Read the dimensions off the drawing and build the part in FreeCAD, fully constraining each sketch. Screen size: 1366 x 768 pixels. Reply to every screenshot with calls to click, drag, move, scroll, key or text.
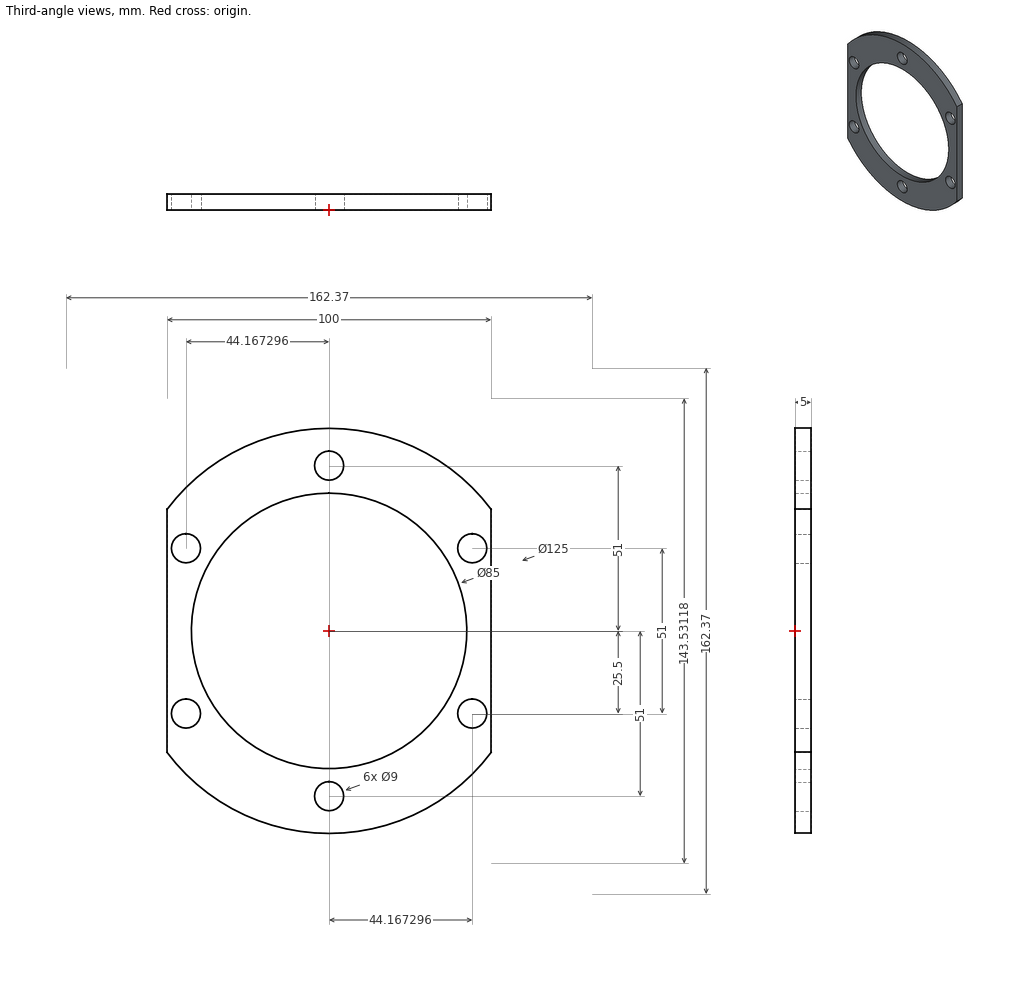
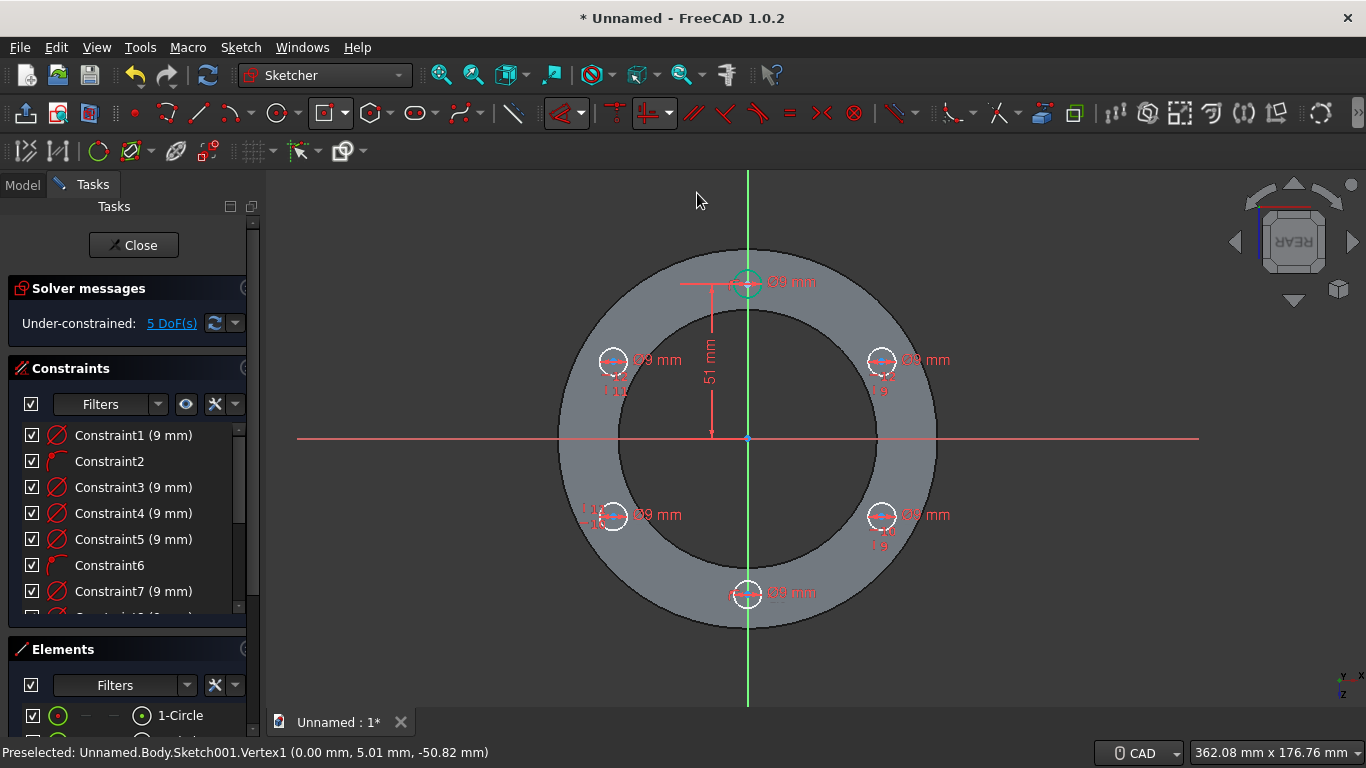
click(748, 595)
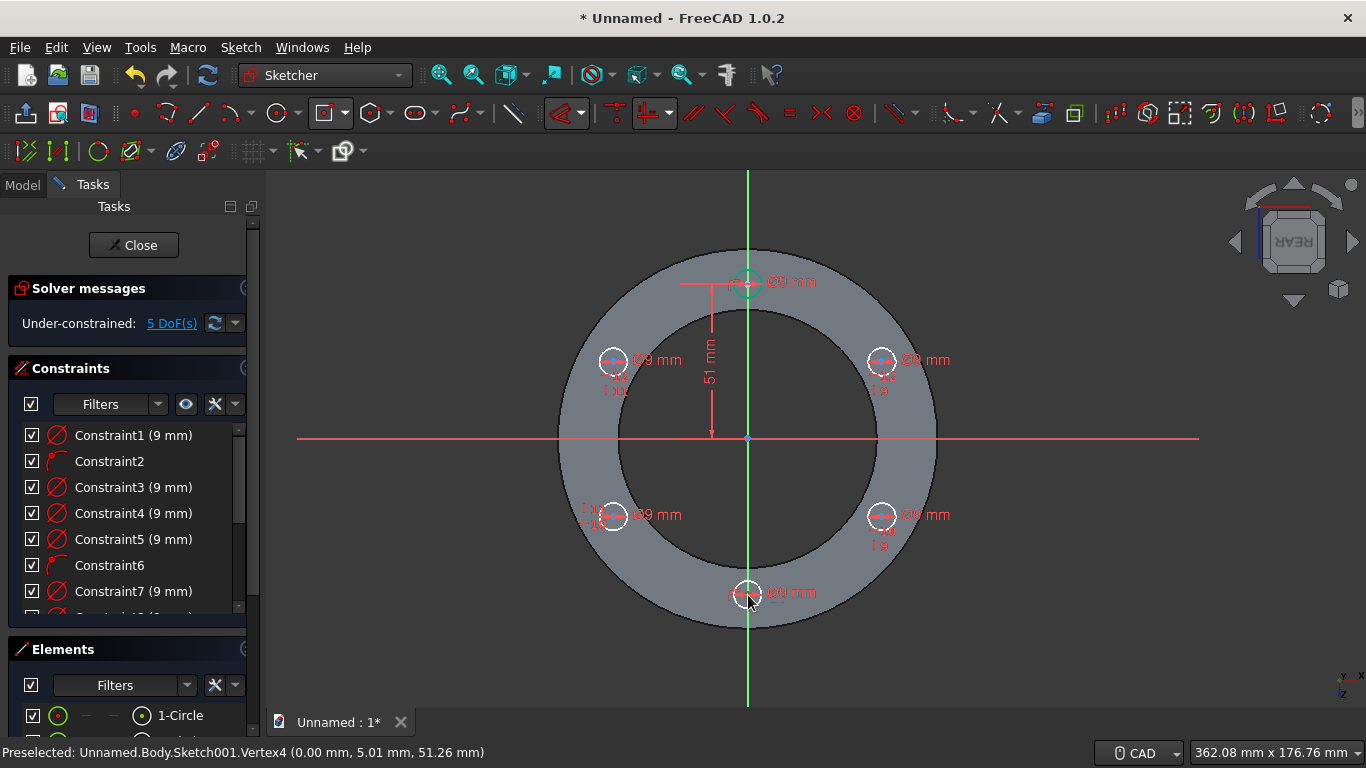
click(584, 114)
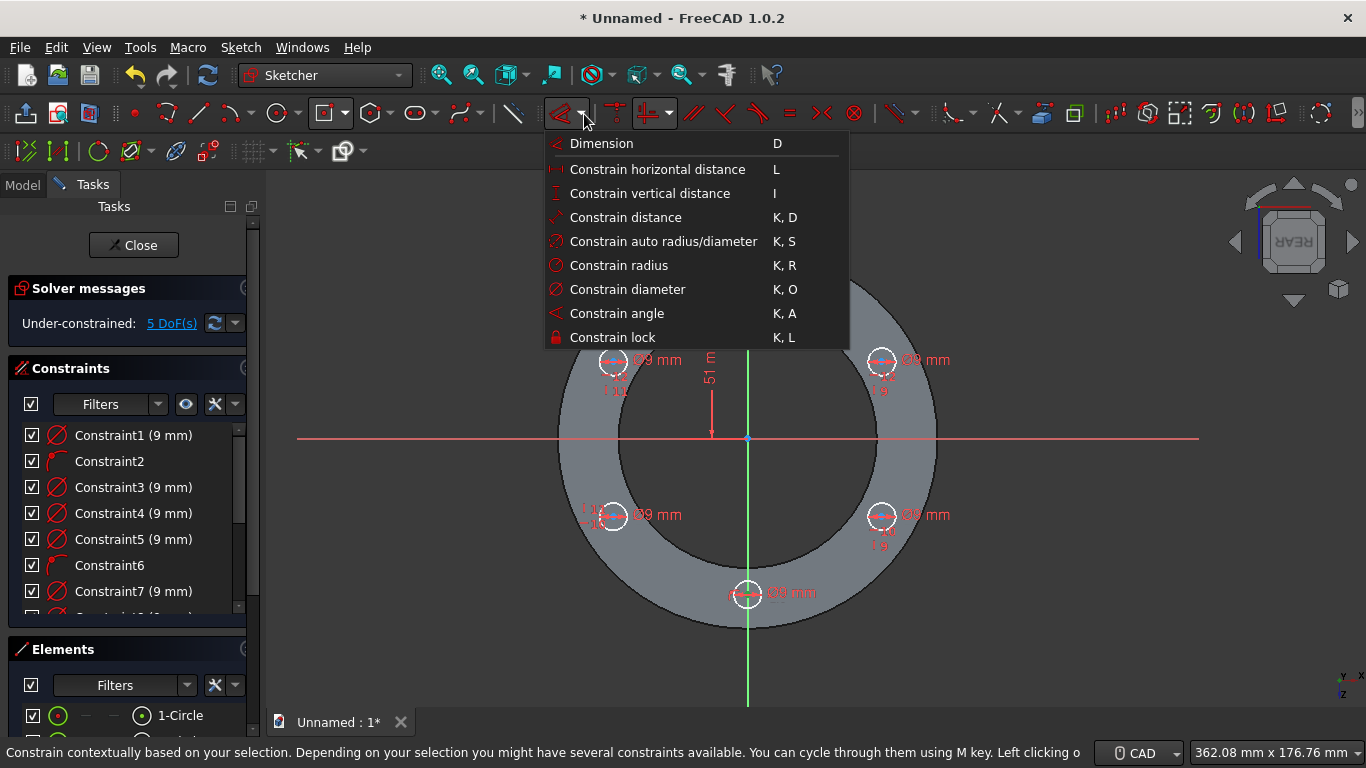
click(697, 193)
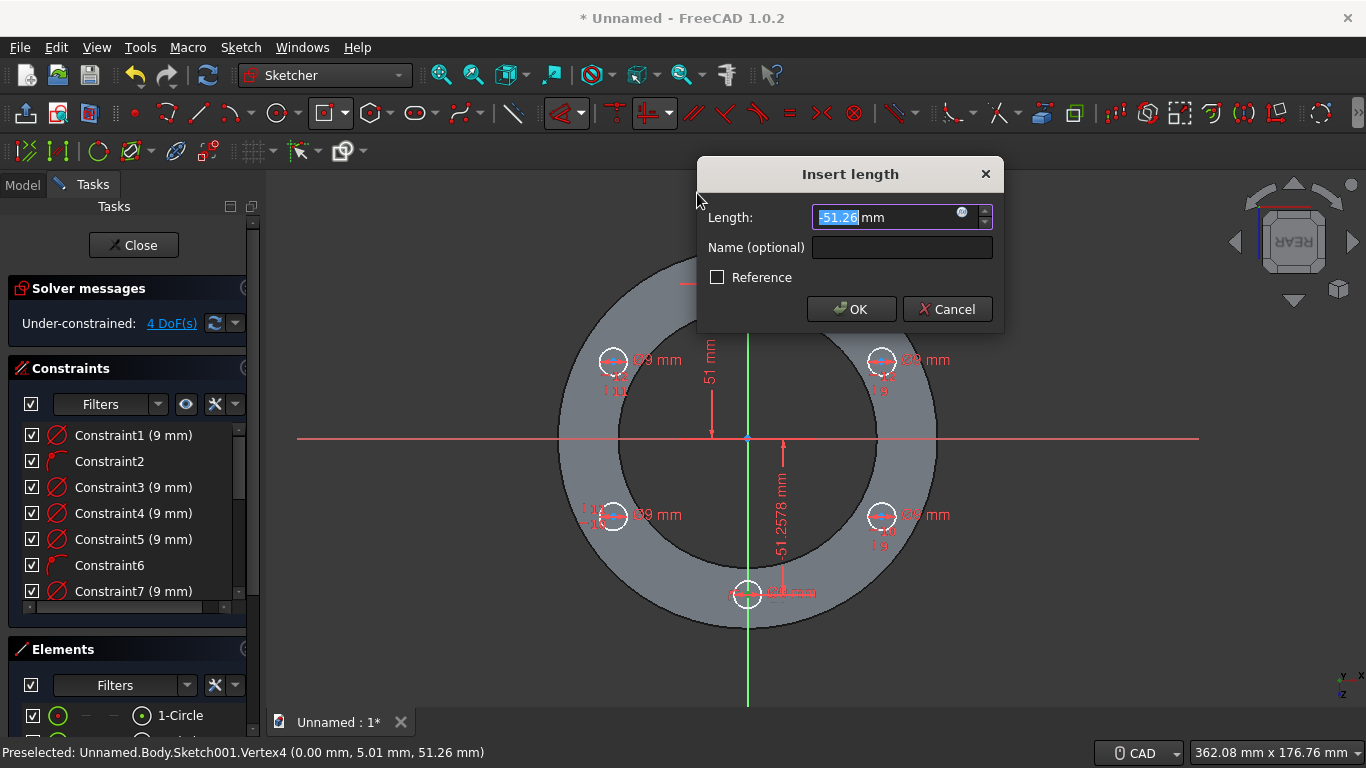
text(-51)
key(Return)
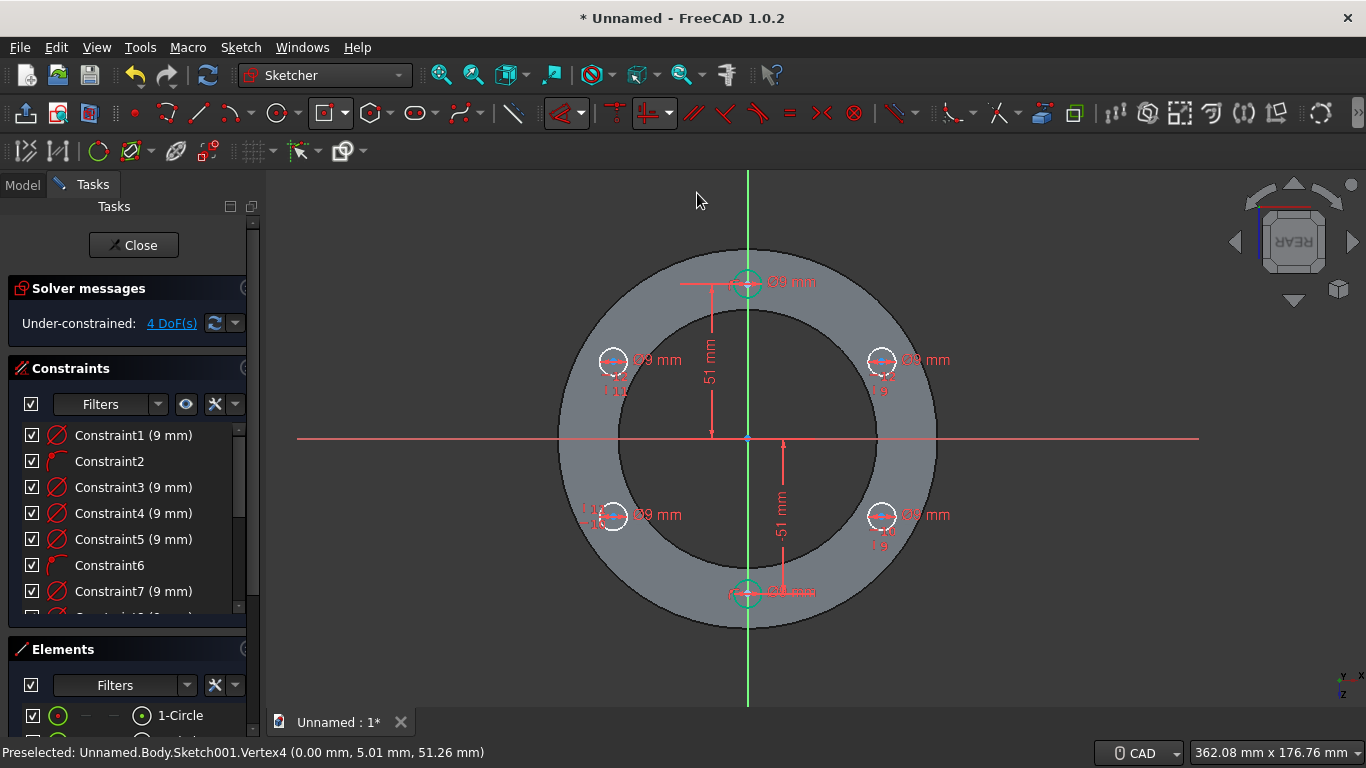
click(882, 362)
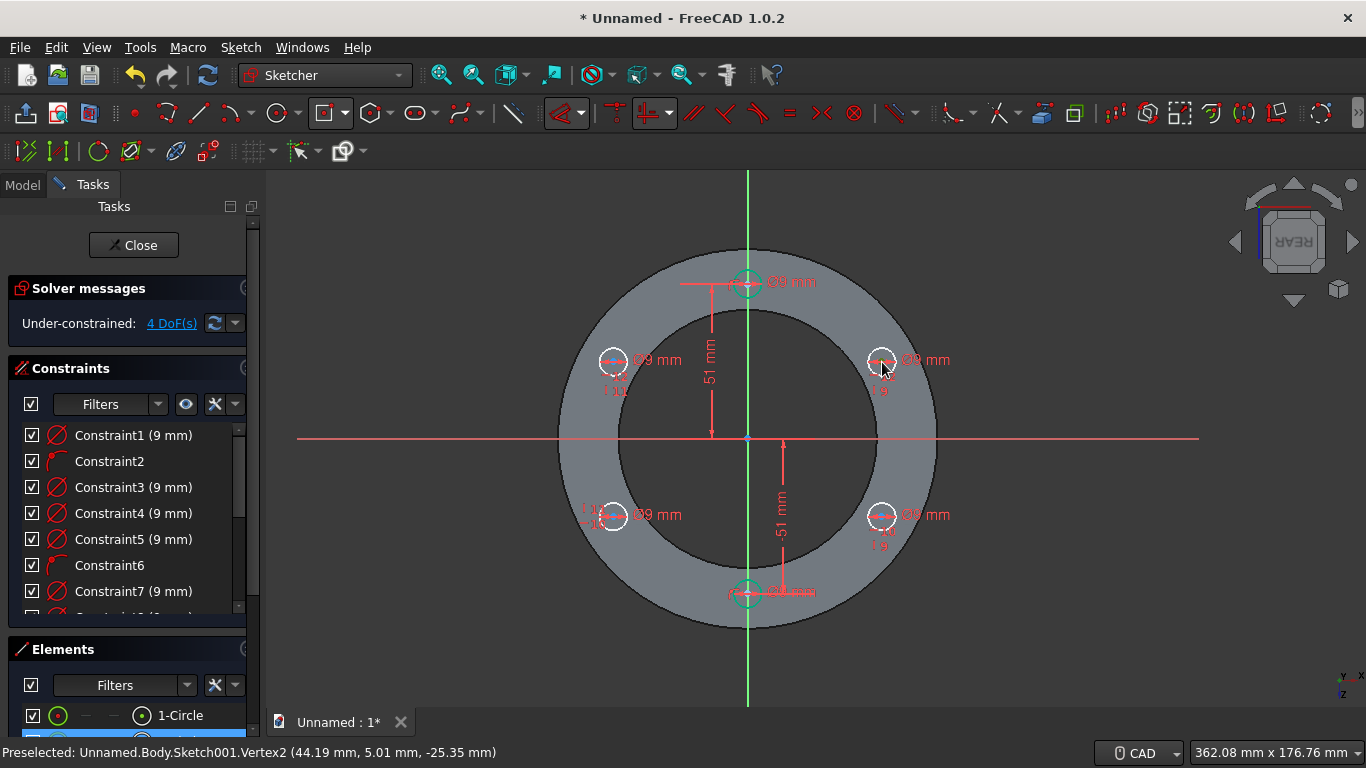
click(882, 517)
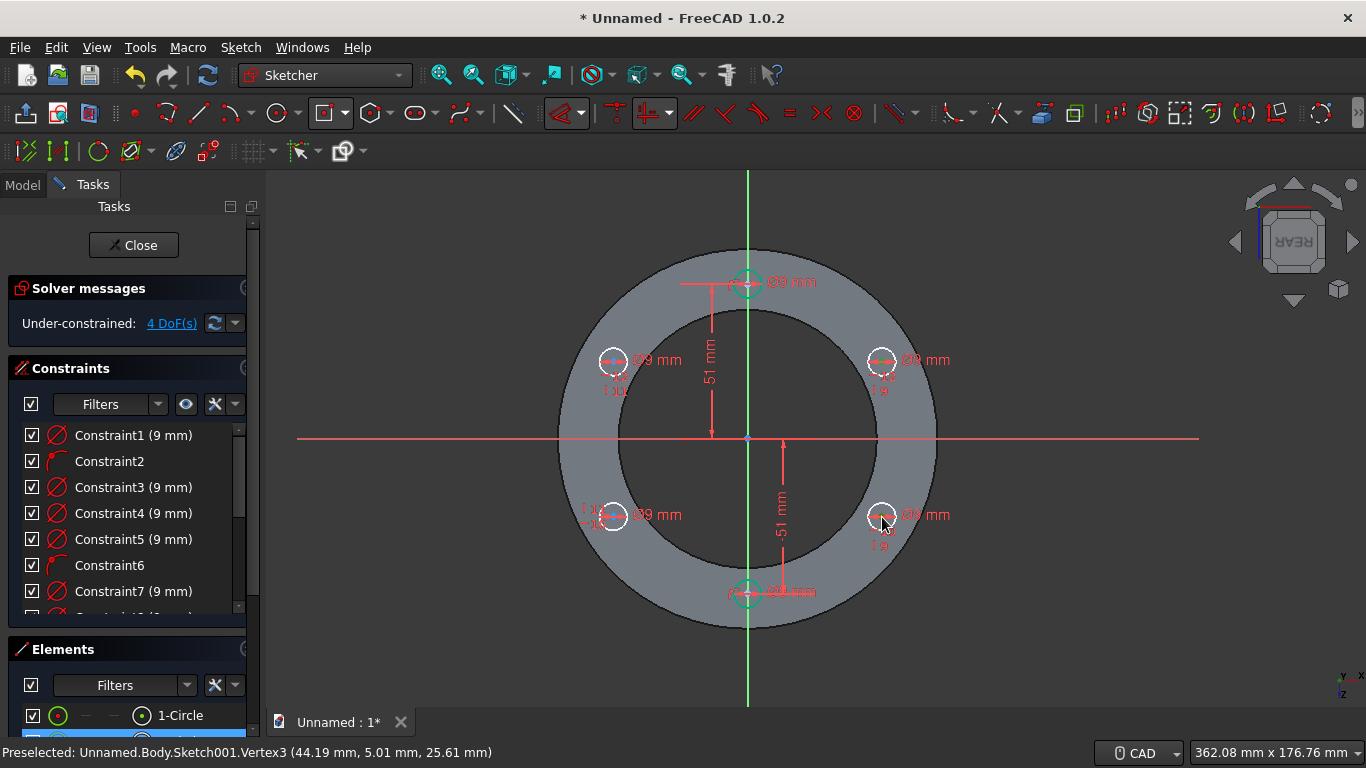
click(584, 114)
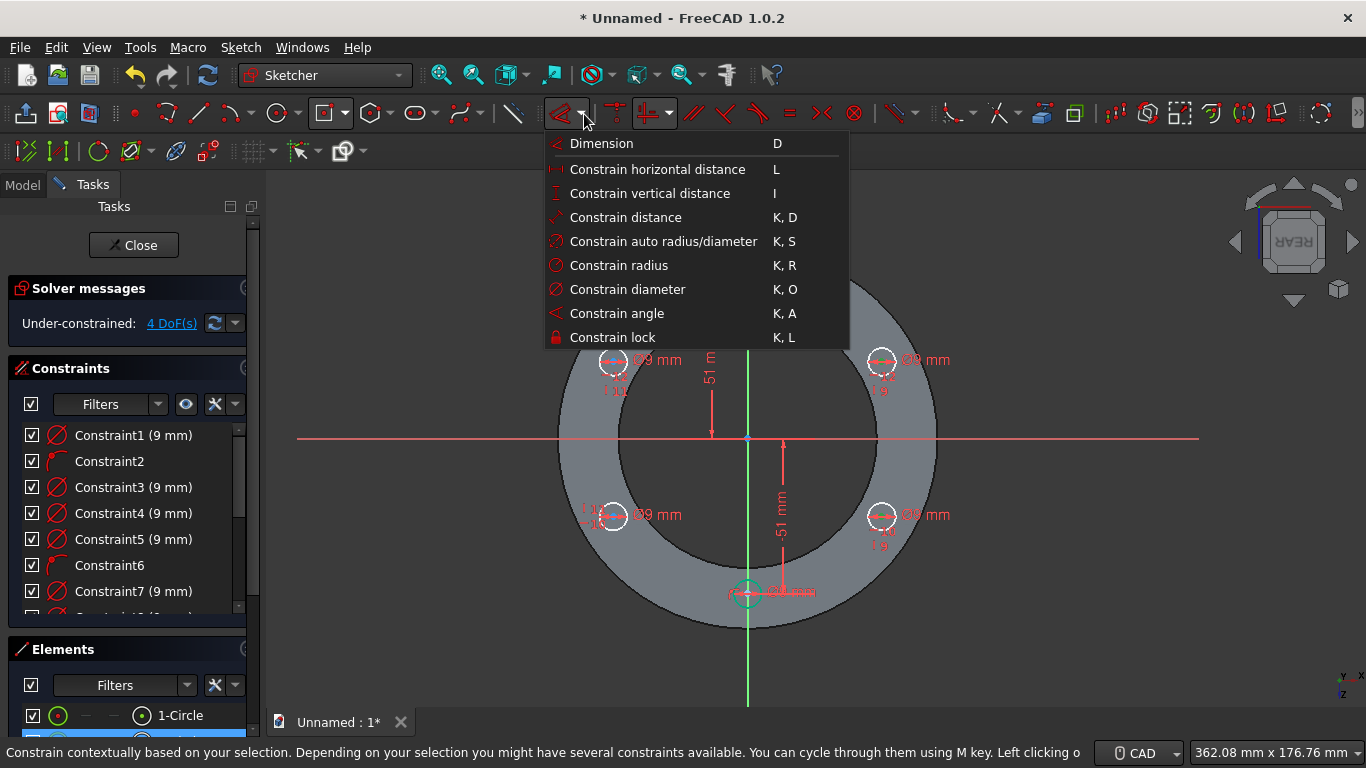
click(697, 193)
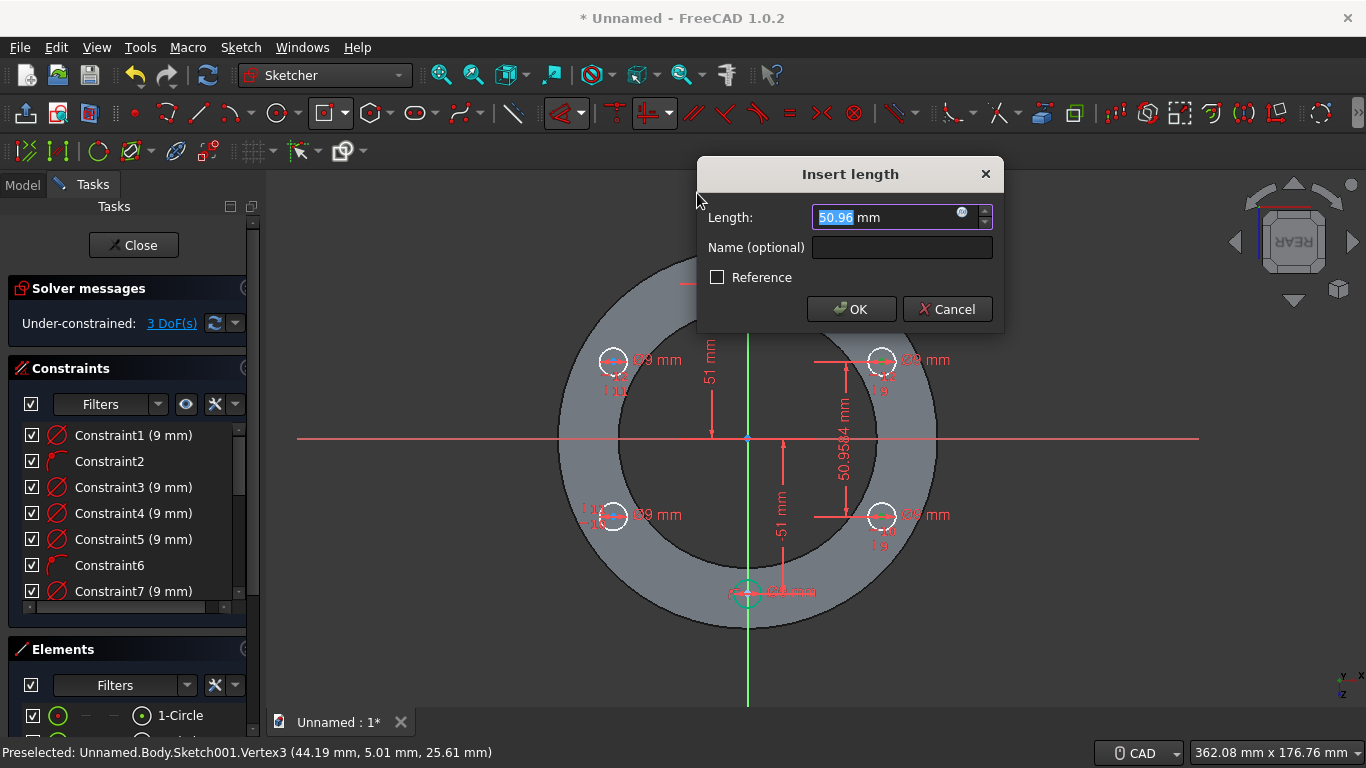
text(51)
key(Return)